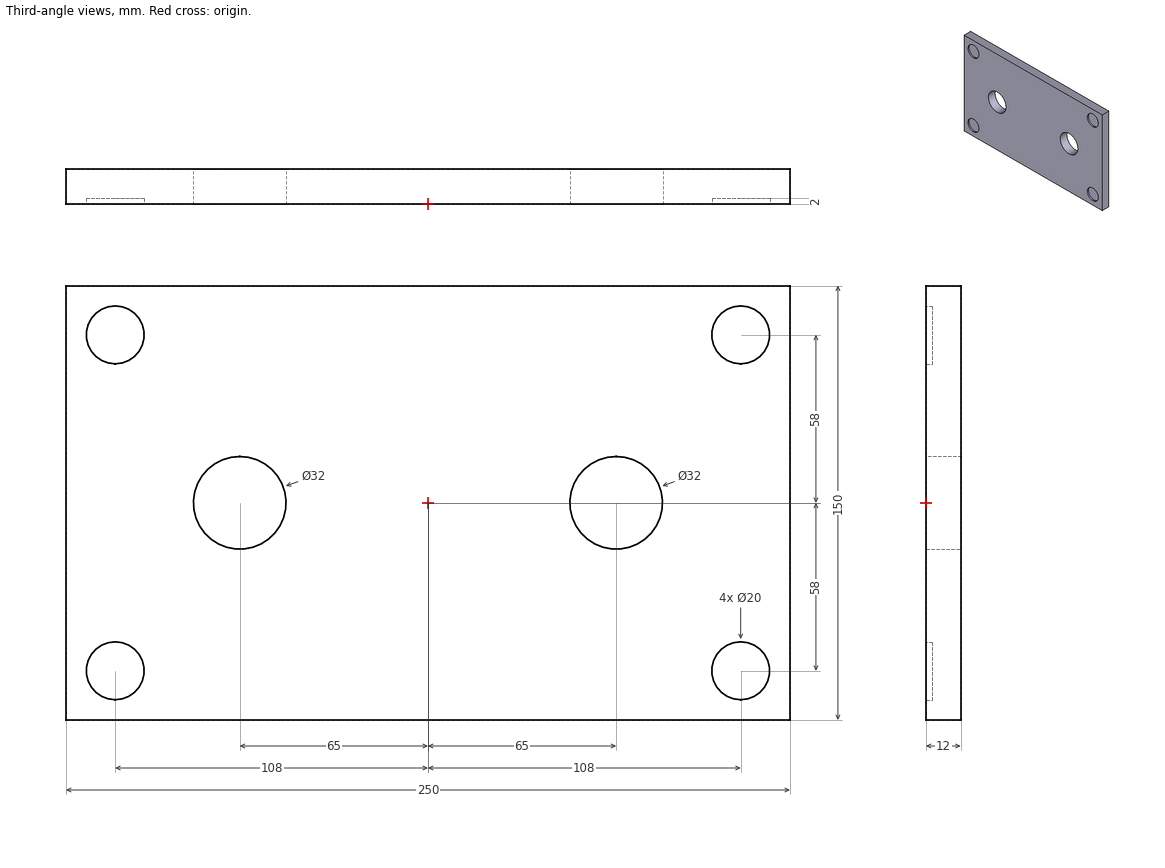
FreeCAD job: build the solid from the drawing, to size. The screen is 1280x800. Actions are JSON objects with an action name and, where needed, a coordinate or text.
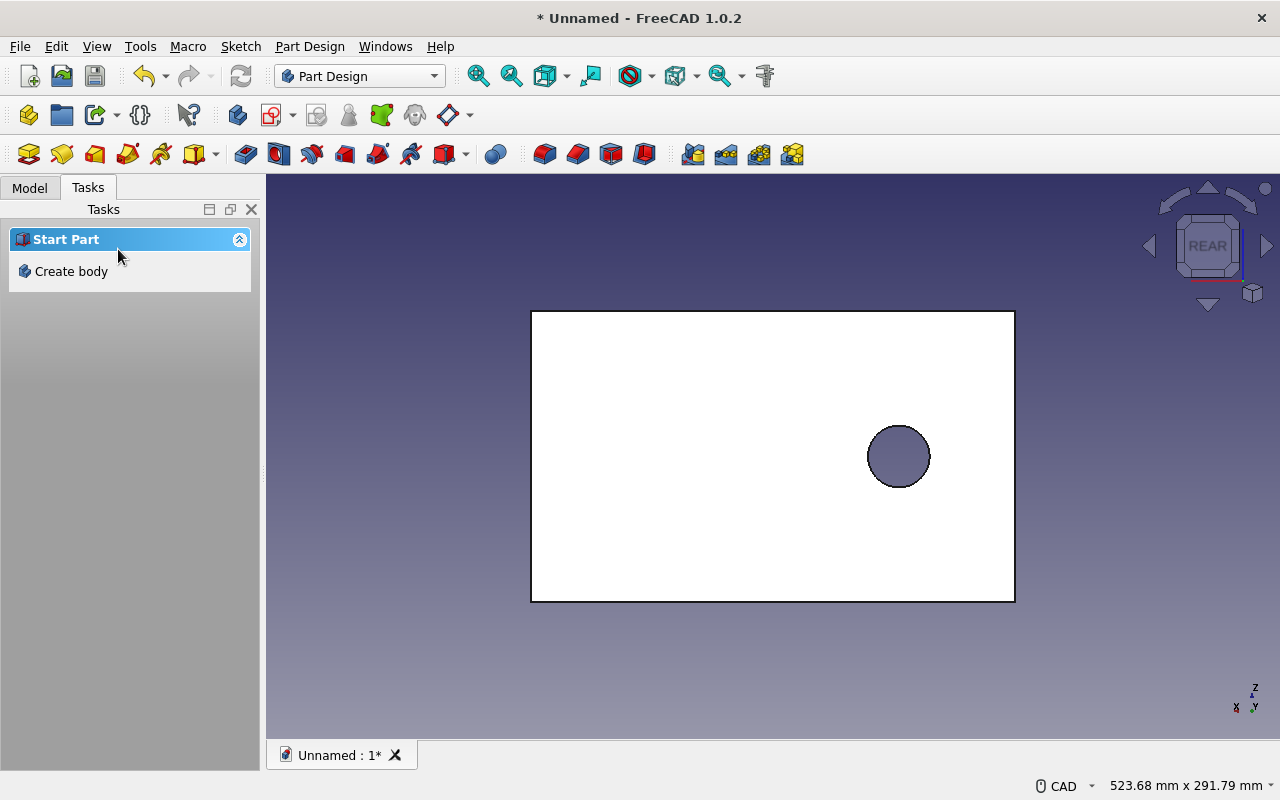
{"action": "left_click", "coordinate": [704, 455]}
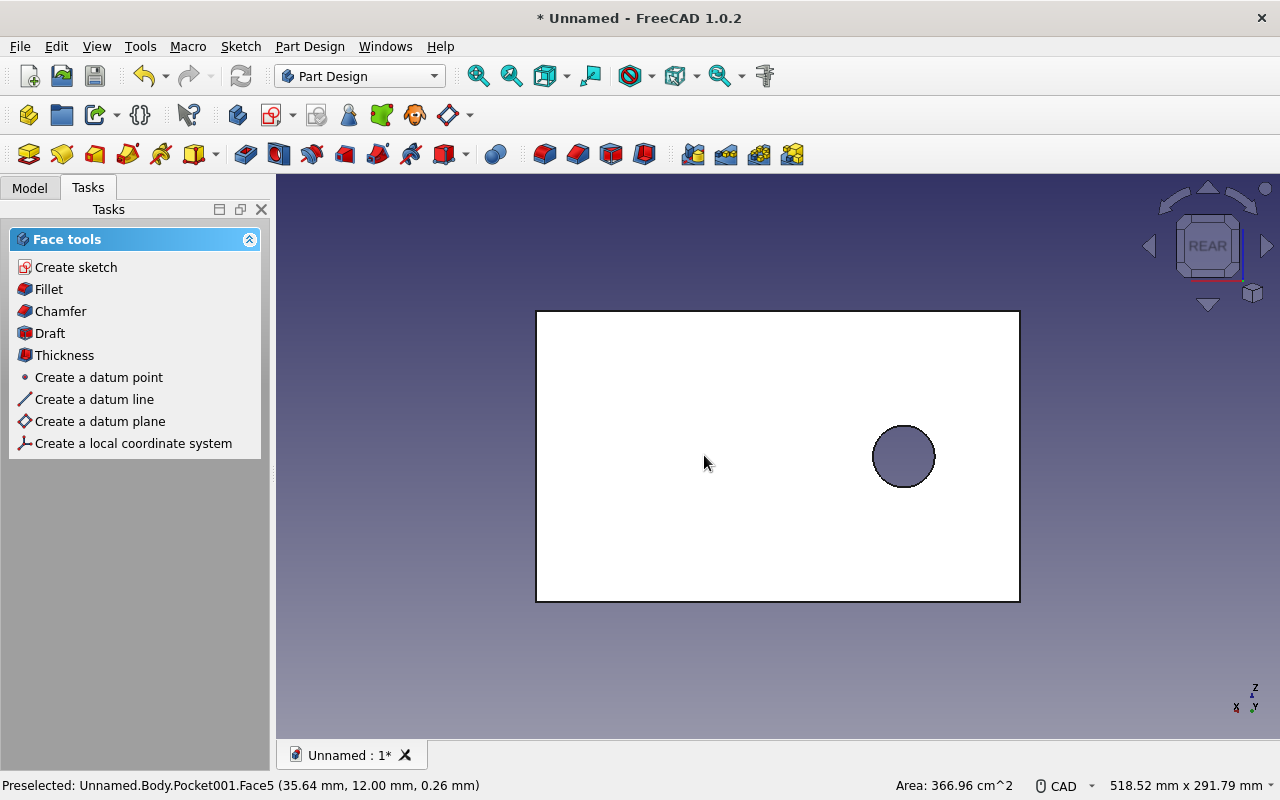
{"action": "left_click", "coordinate": [270, 116]}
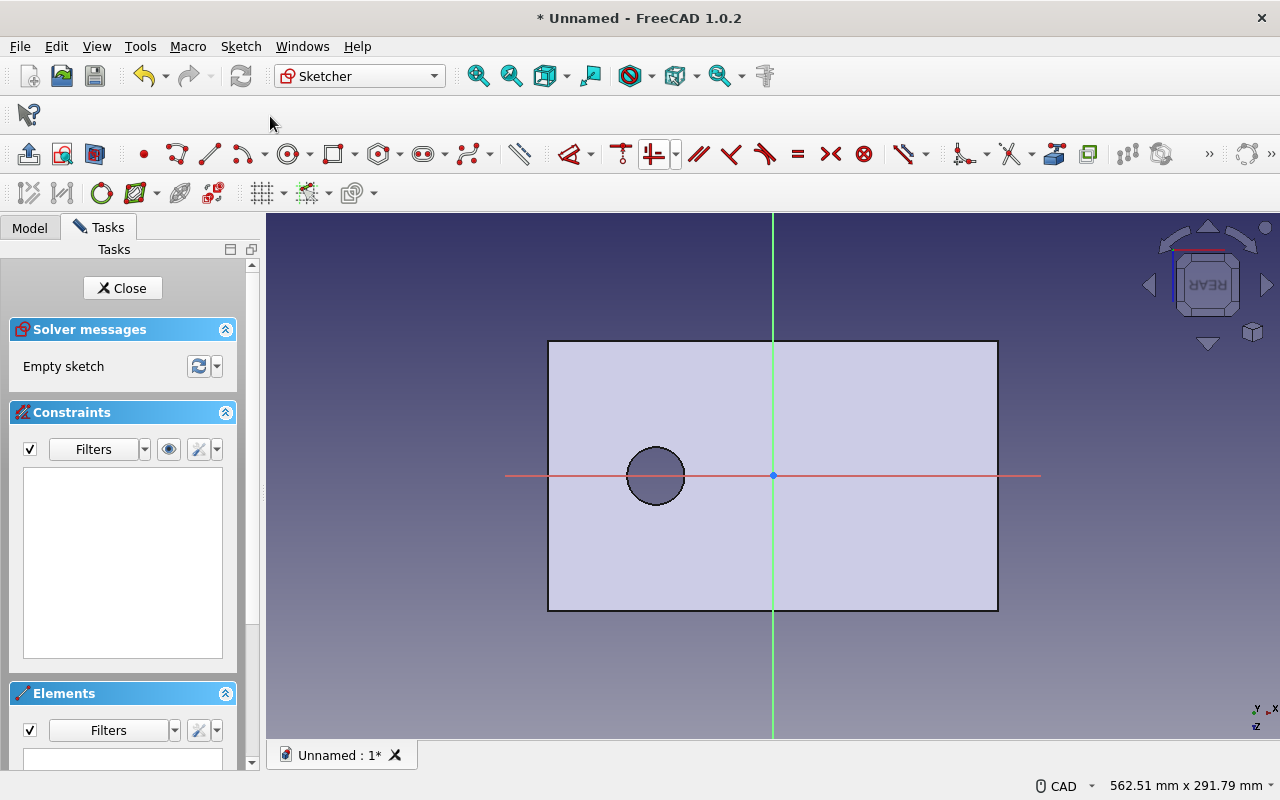
{"action": "scroll", "coordinate": [927, 476], "scroll_direction": "up", "scroll_amount": 9}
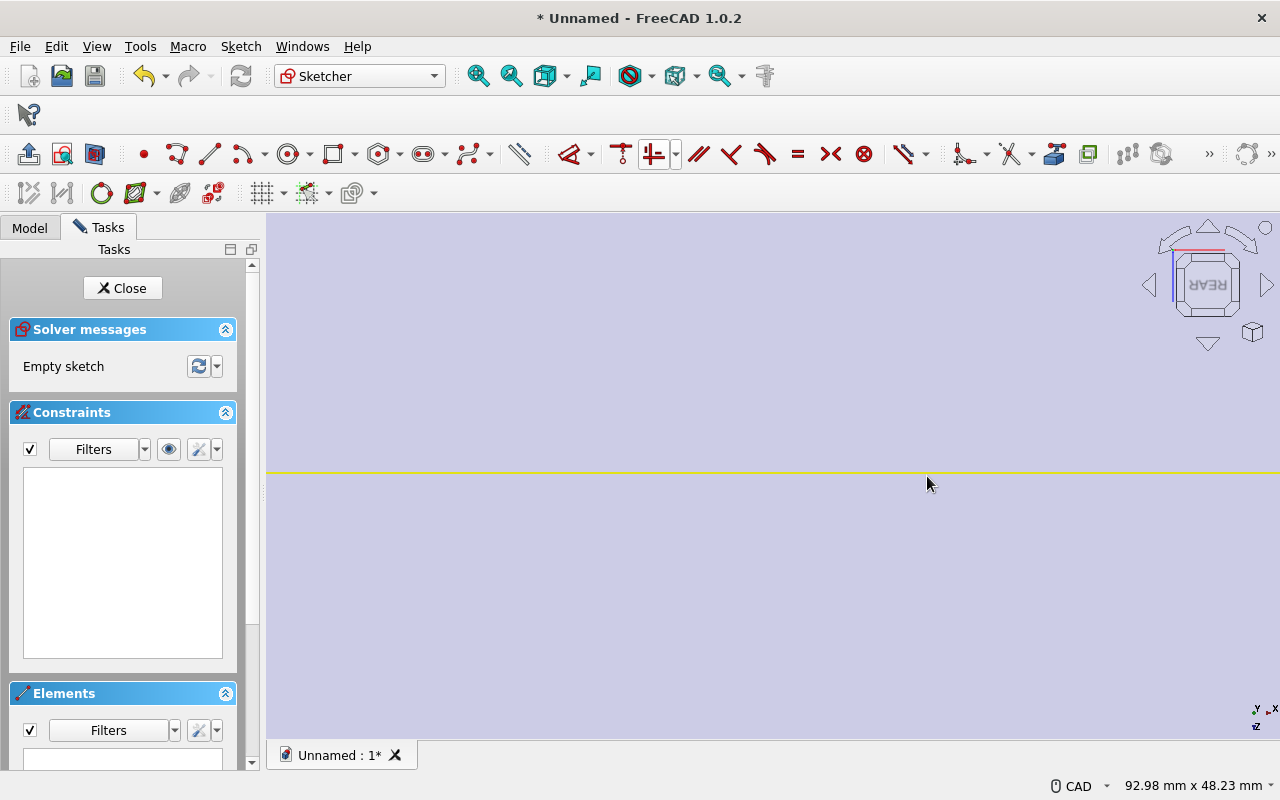
{"action": "key", "text": "g c"}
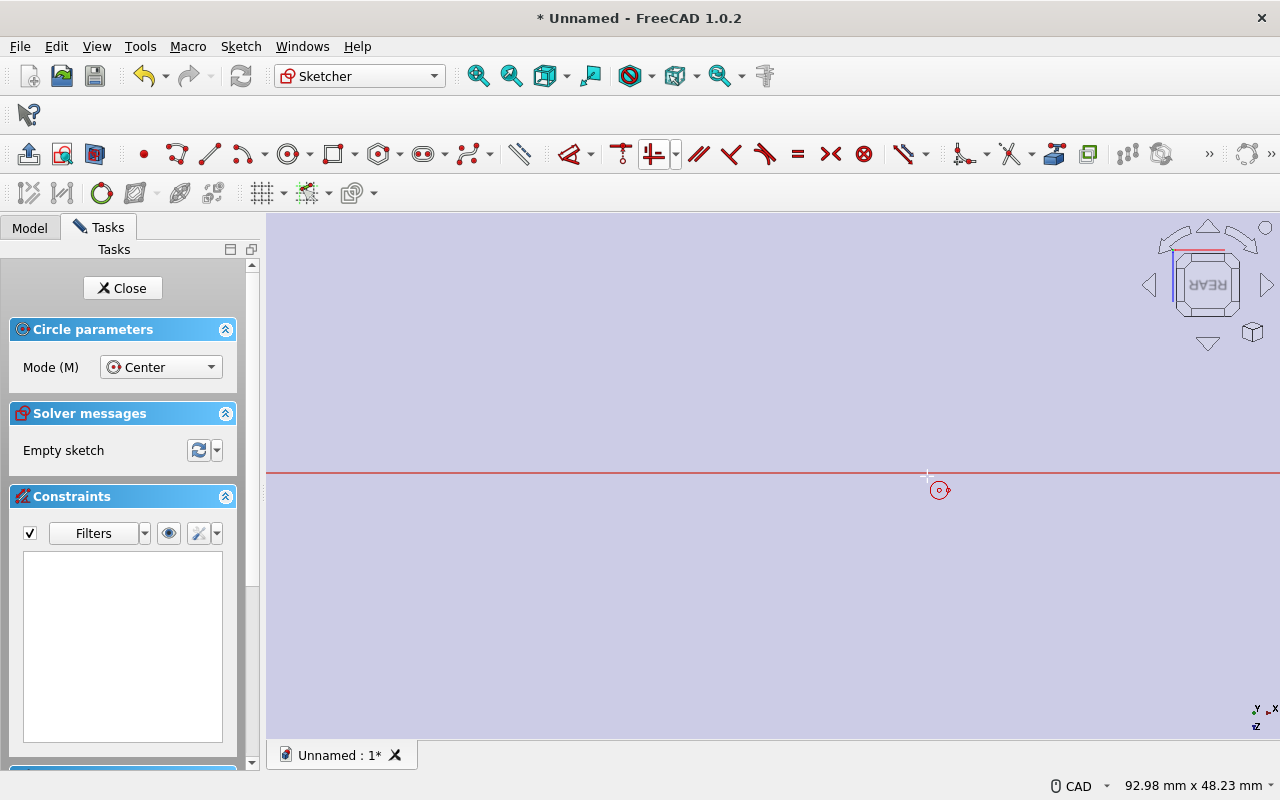
{"action": "left_click", "coordinate": [701, 473]}
{"action": "mouse_move", "coordinate": [824, 350]}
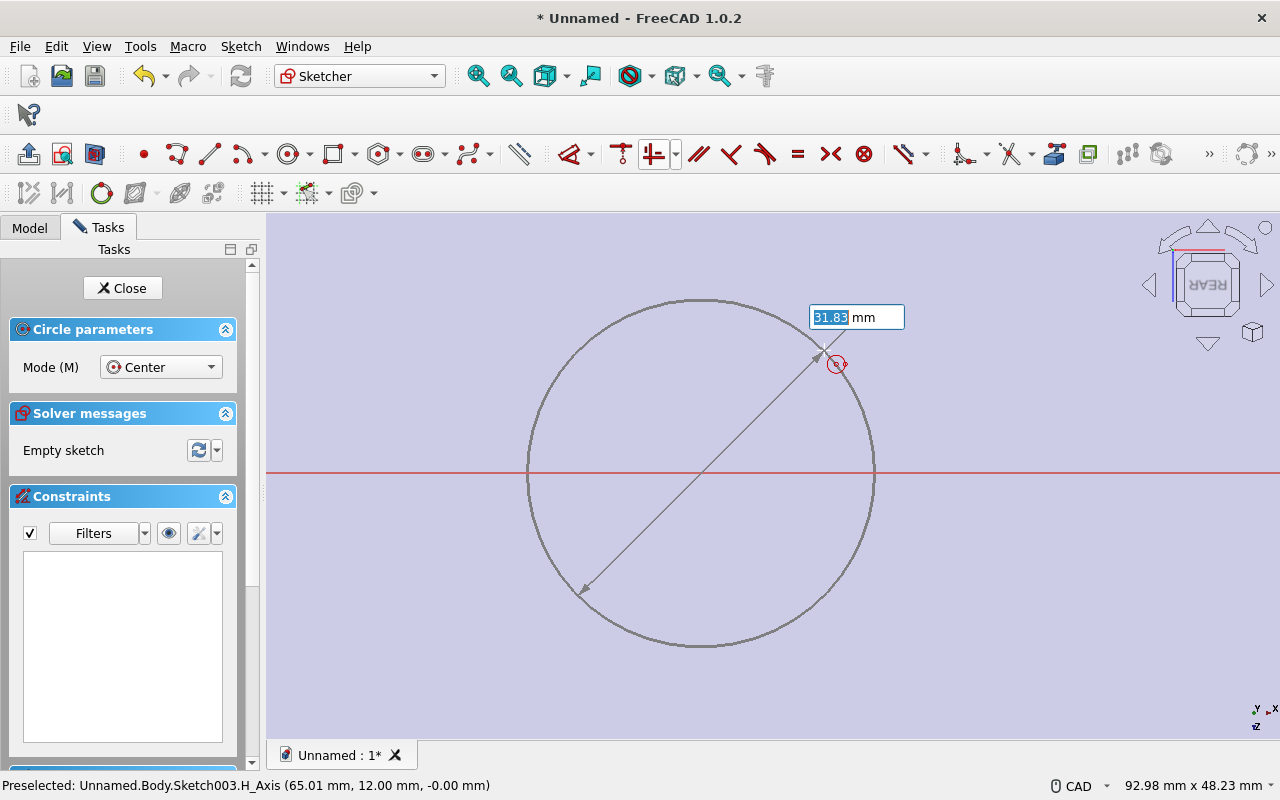
{"action": "type", "text": "32"}
{"action": "key", "text": "Return"}
{"action": "key", "text": "Escape"}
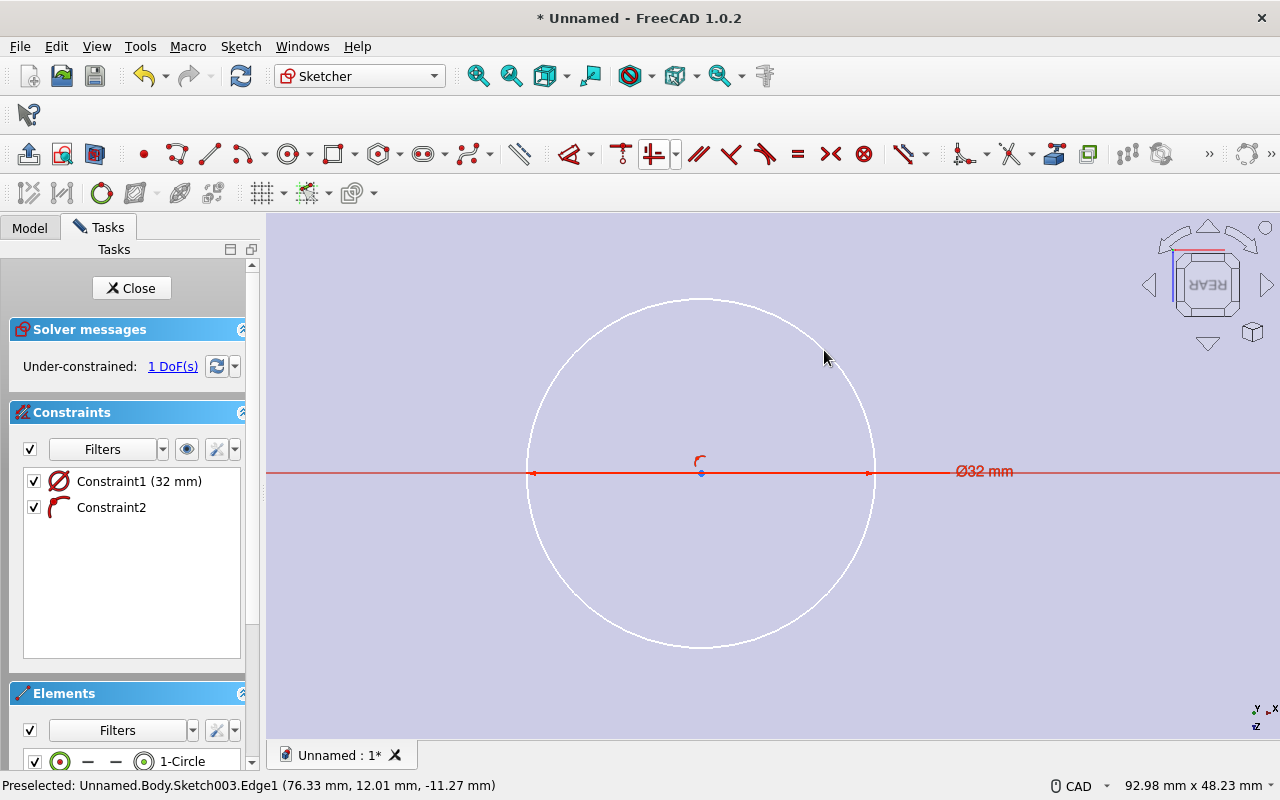
{"action": "left_click", "coordinate": [568, 154]}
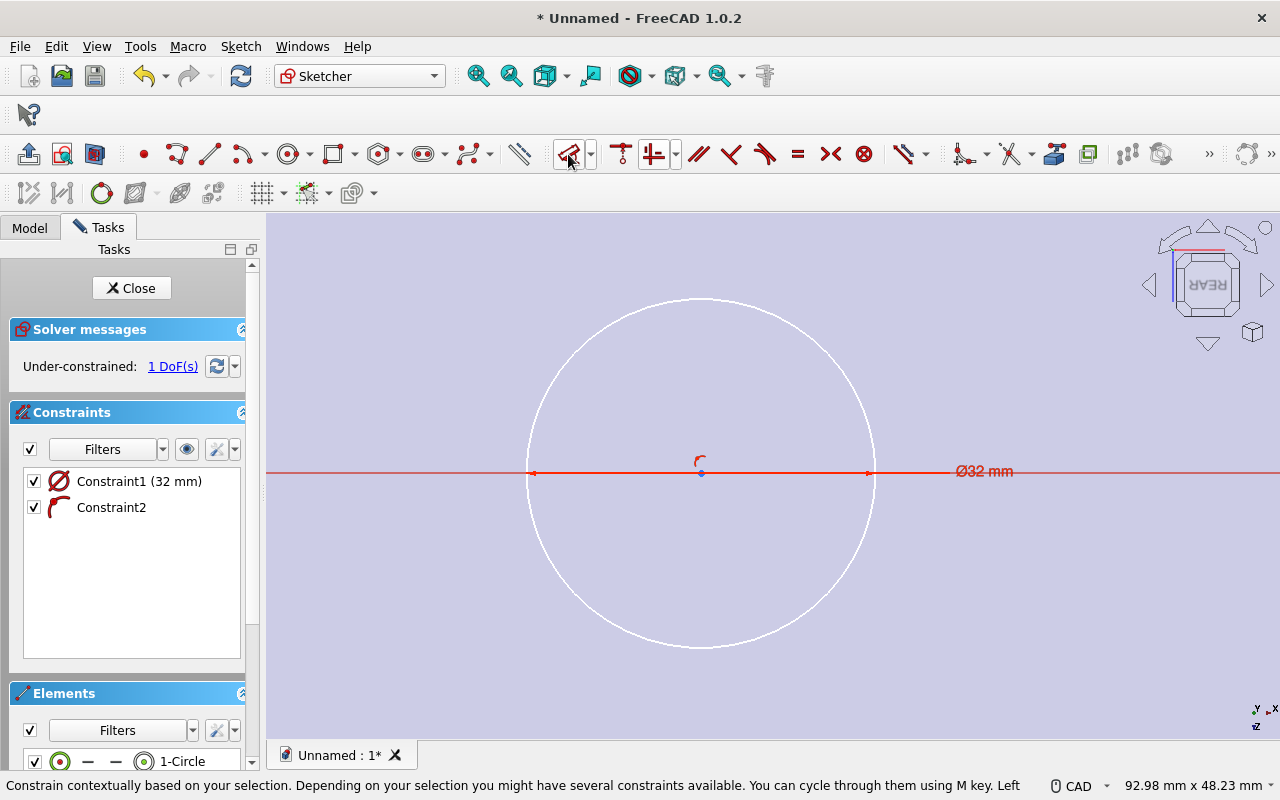
{"action": "left_click", "coordinate": [701, 473]}
{"action": "left_click", "coordinate": [497, 507]}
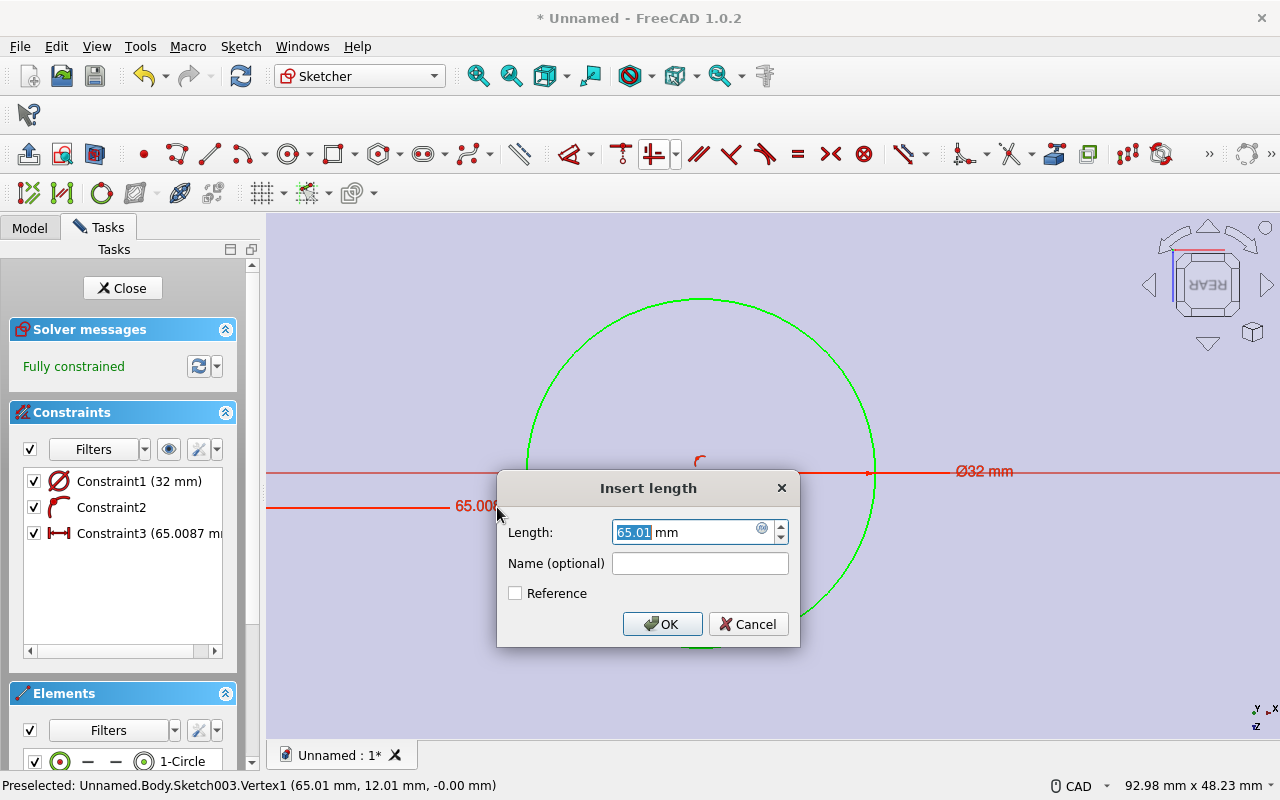
{"action": "type", "text": "65"}
{"action": "key", "text": "Return"}
{"action": "key", "text": "Escape"}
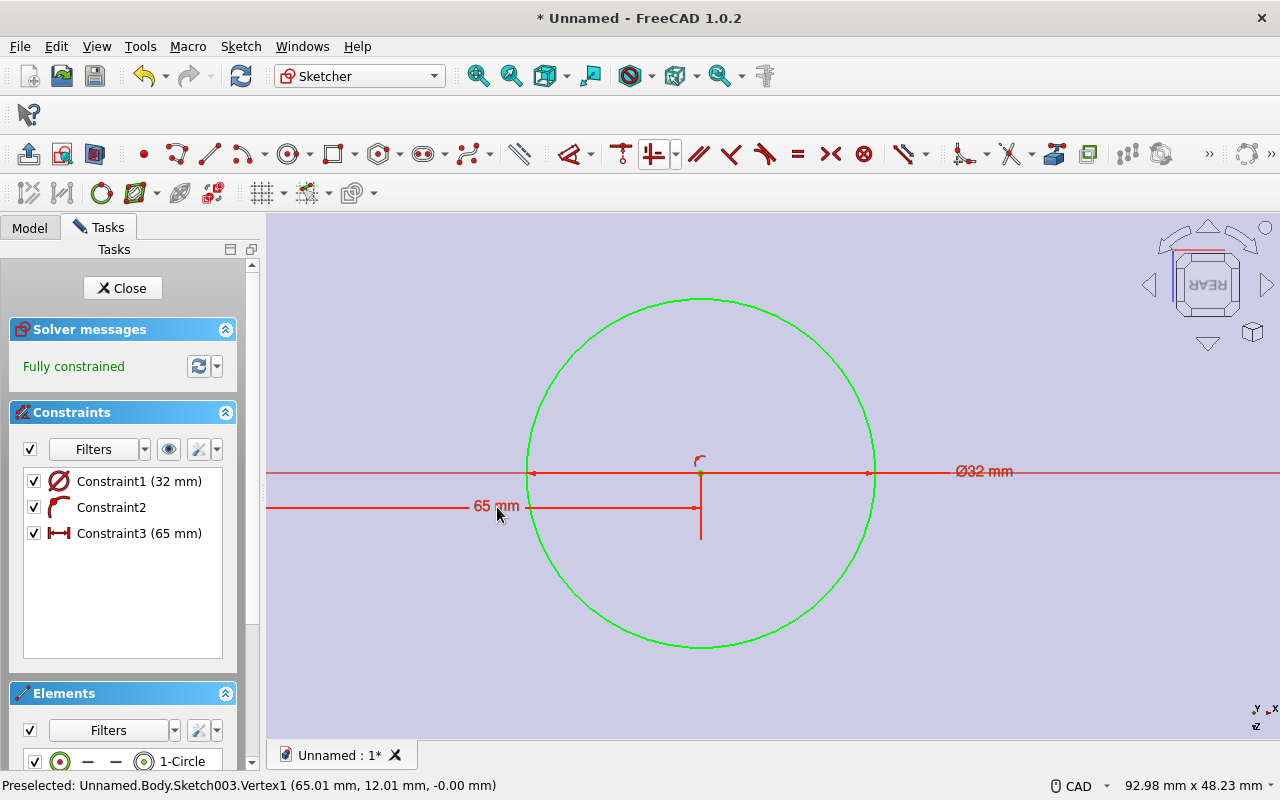
{"action": "left_click", "coordinate": [123, 288]}